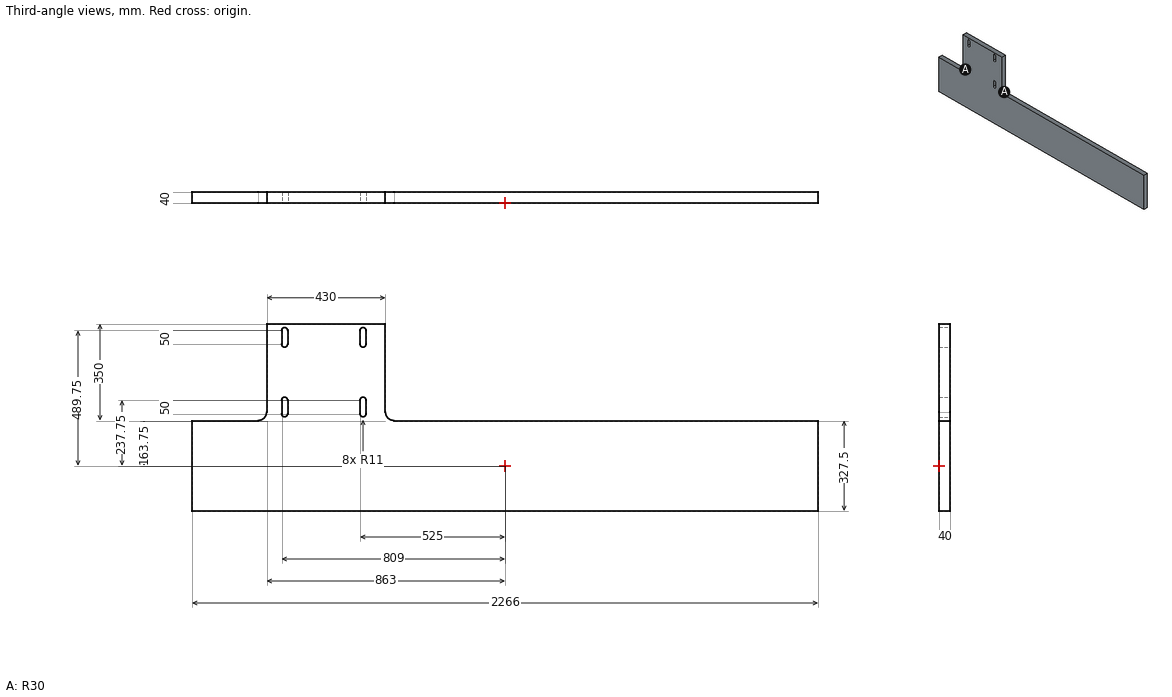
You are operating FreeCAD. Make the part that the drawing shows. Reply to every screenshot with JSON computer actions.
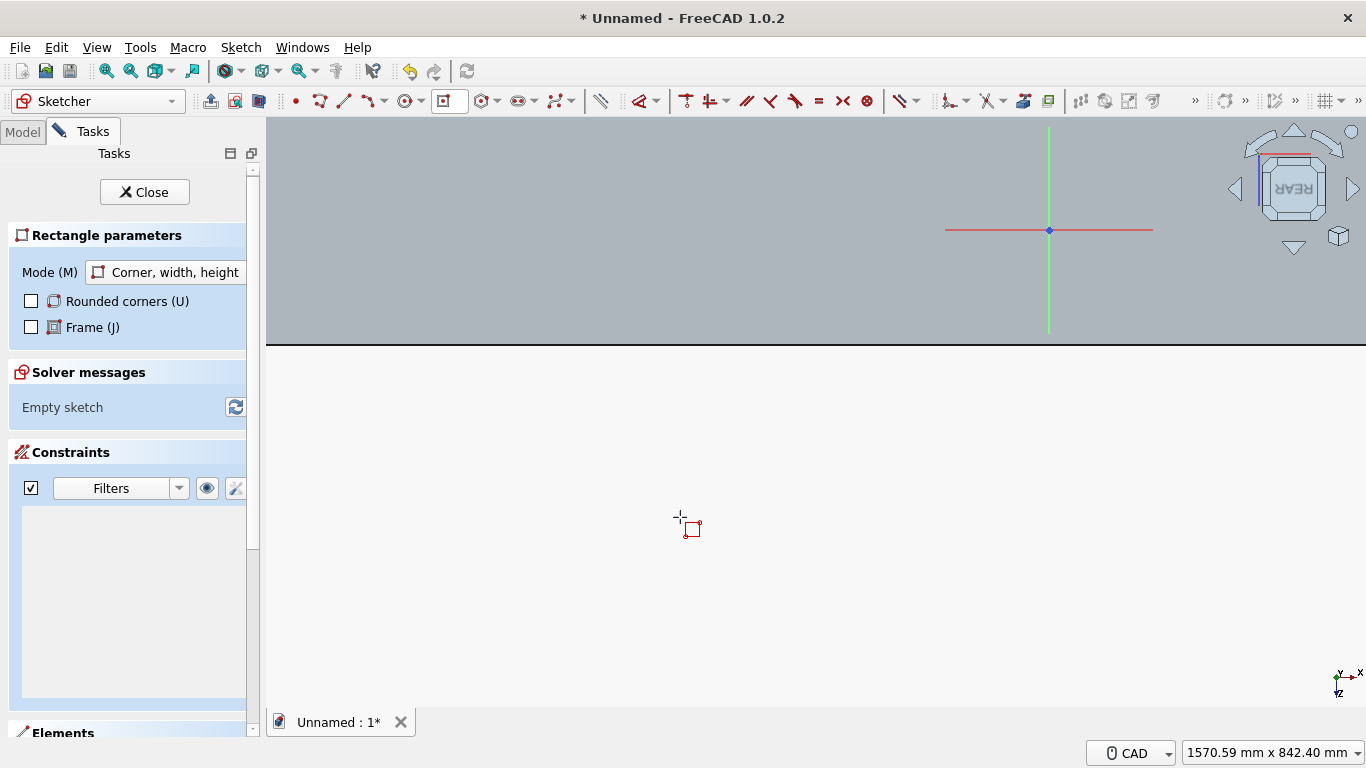
{"action": "left_click", "coordinate": [445, 345]}
{"action": "mouse_move", "coordinate": [746, 590]}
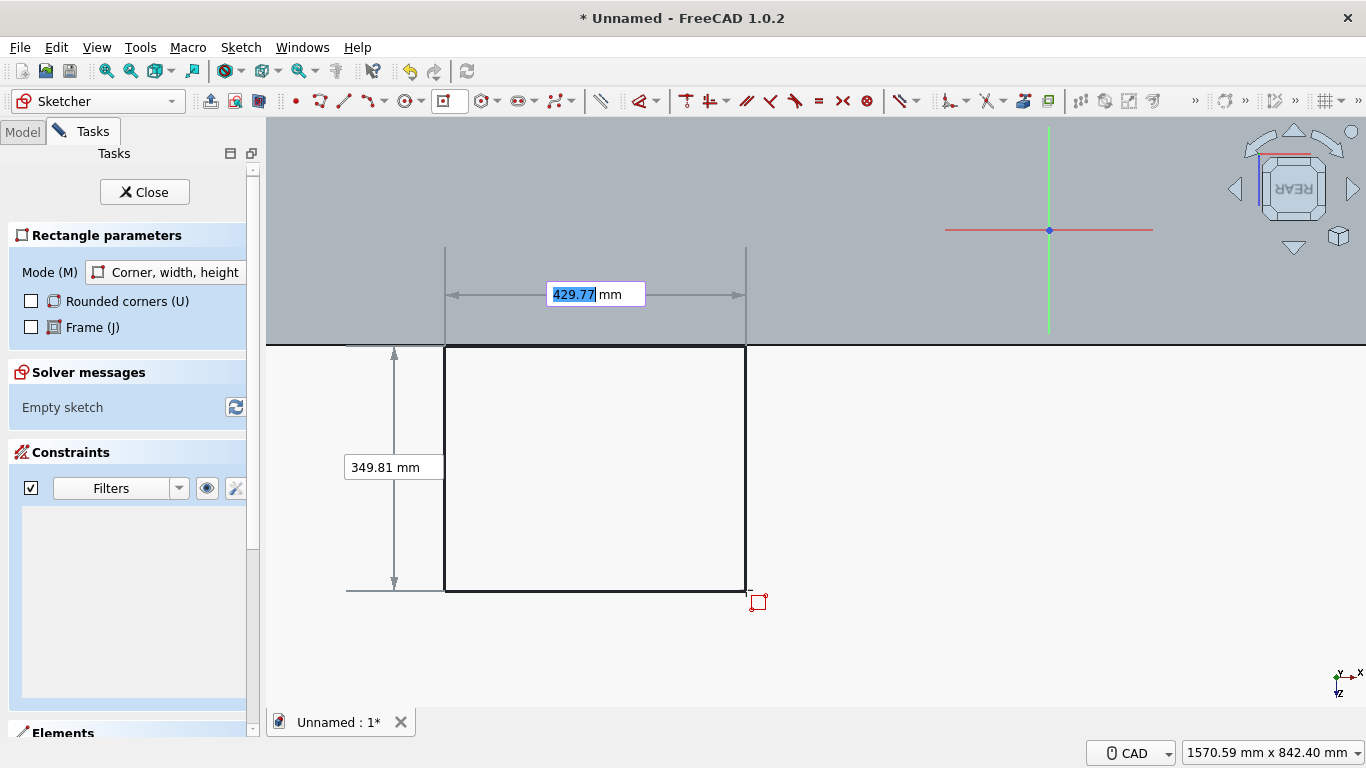
{"action": "type", "text": "430"}
{"action": "key", "text": "Tab"}
{"action": "type", "text": "350"}
{"action": "key", "text": "Return"}
{"action": "key", "text": "Escape"}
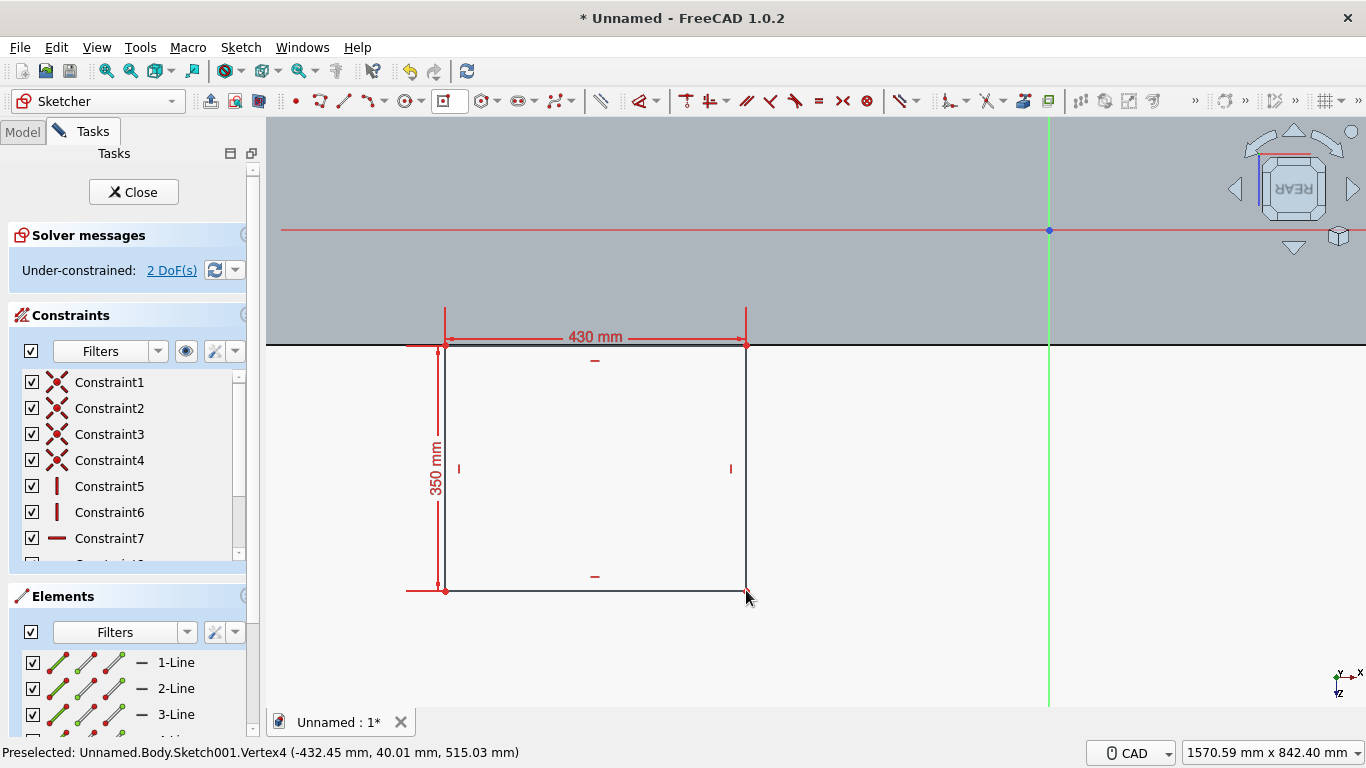
{"action": "left_click", "coordinate": [640, 102]}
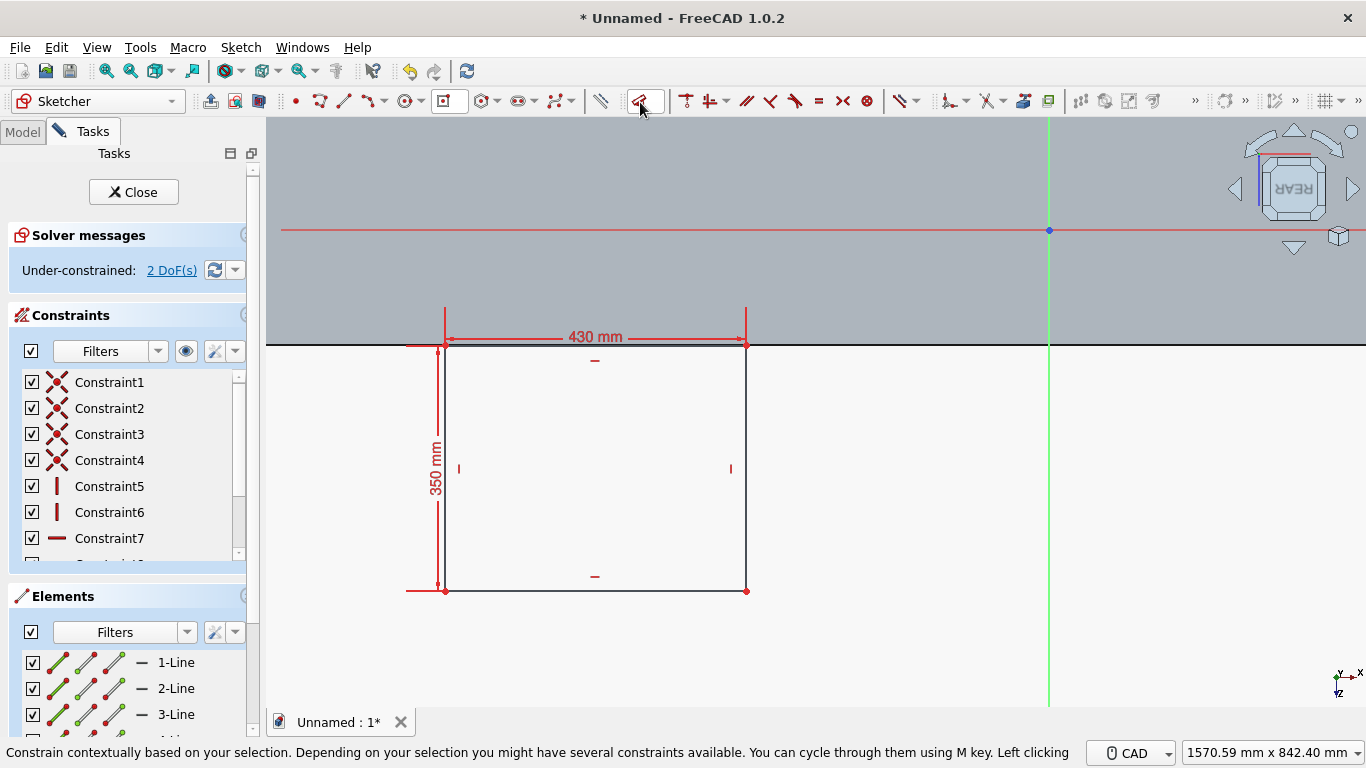
{"action": "left_click", "coordinate": [445, 346]}
{"action": "left_click", "coordinate": [747, 196]}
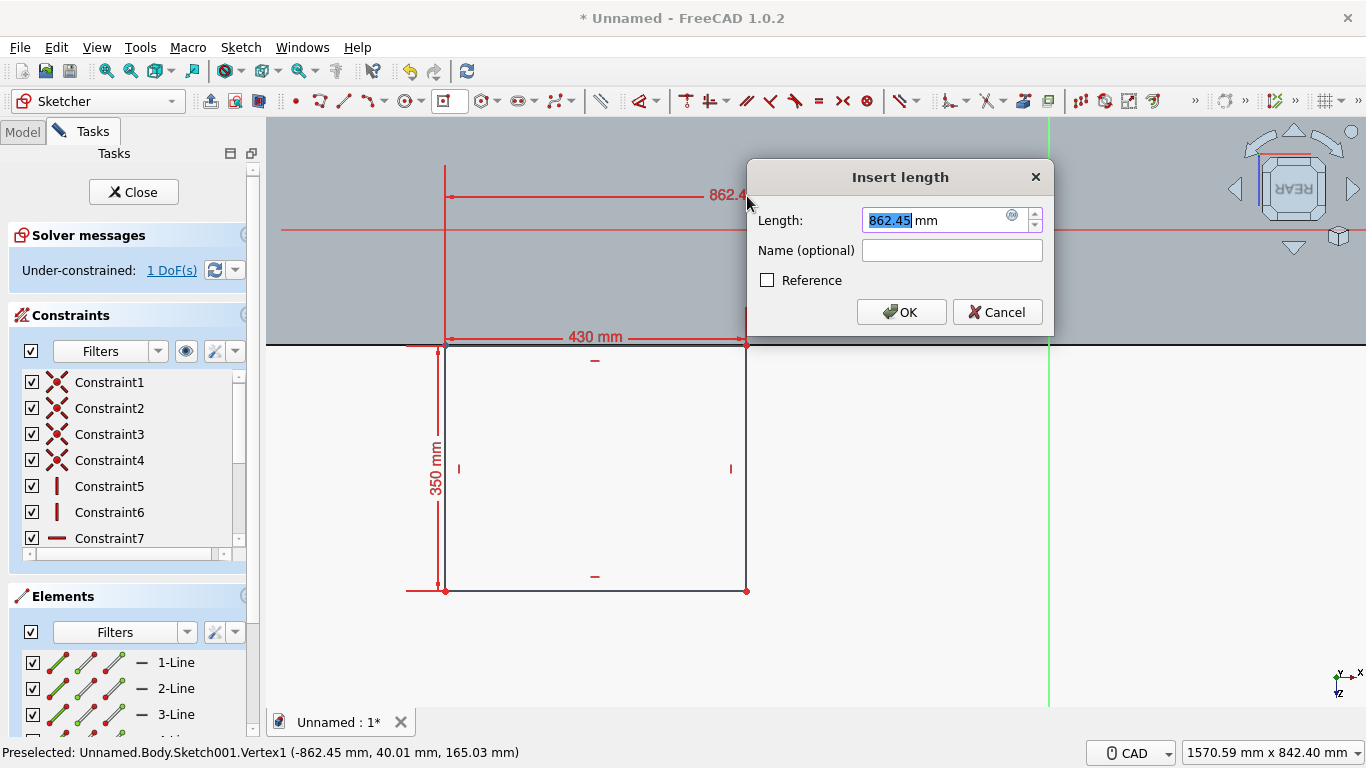
{"action": "type", "text": "863"}
{"action": "key", "text": "Return"}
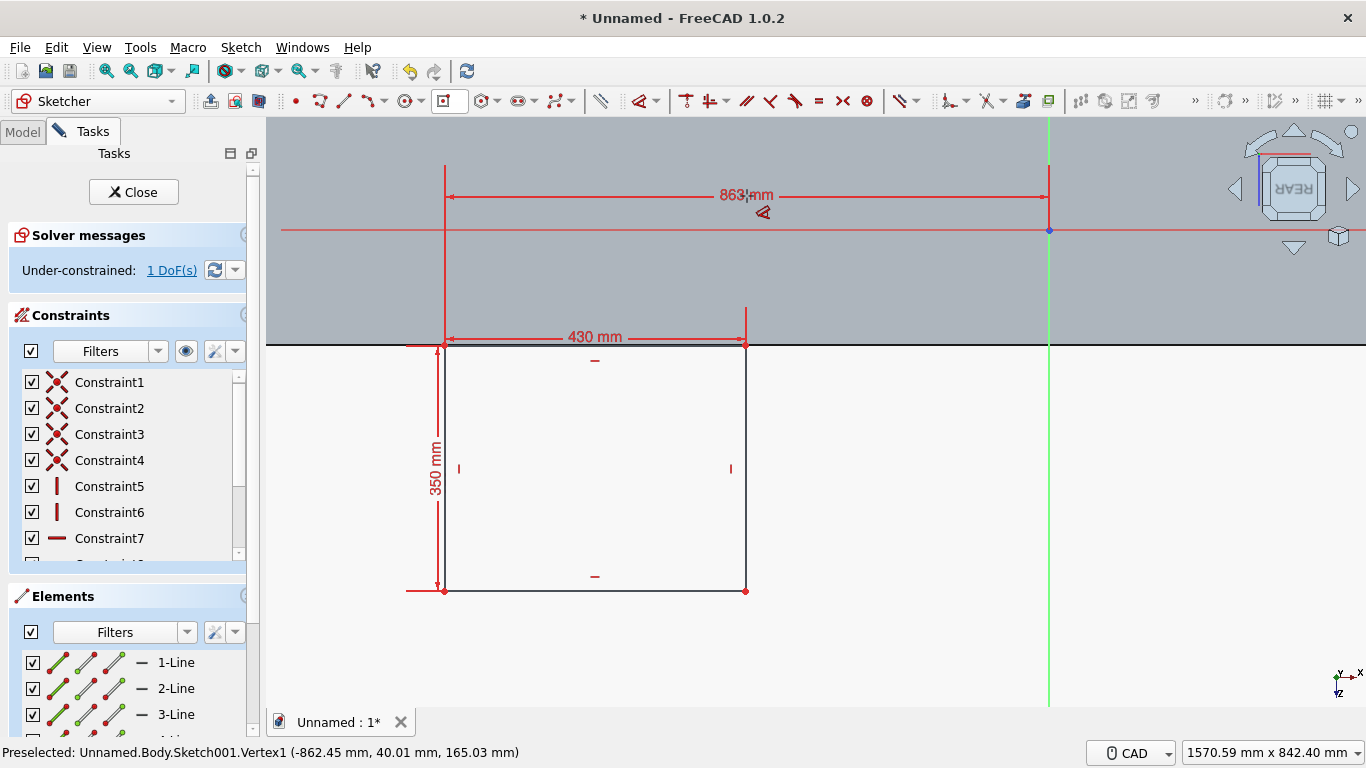
{"action": "left_click", "coordinate": [445, 346]}
{"action": "left_click", "coordinate": [1083, 288]}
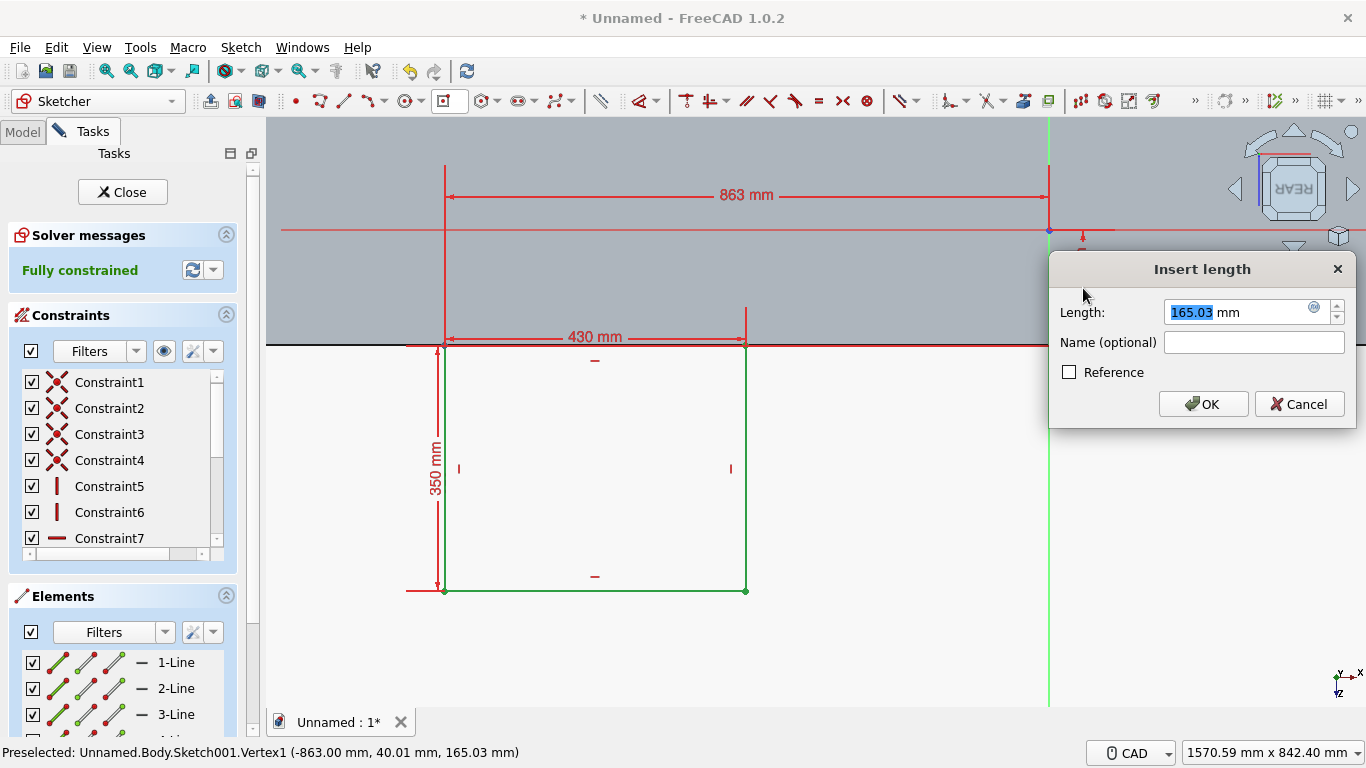
{"action": "type", "text": "163.75"}
{"action": "key", "text": "Return"}
{"action": "key", "text": "Escape"}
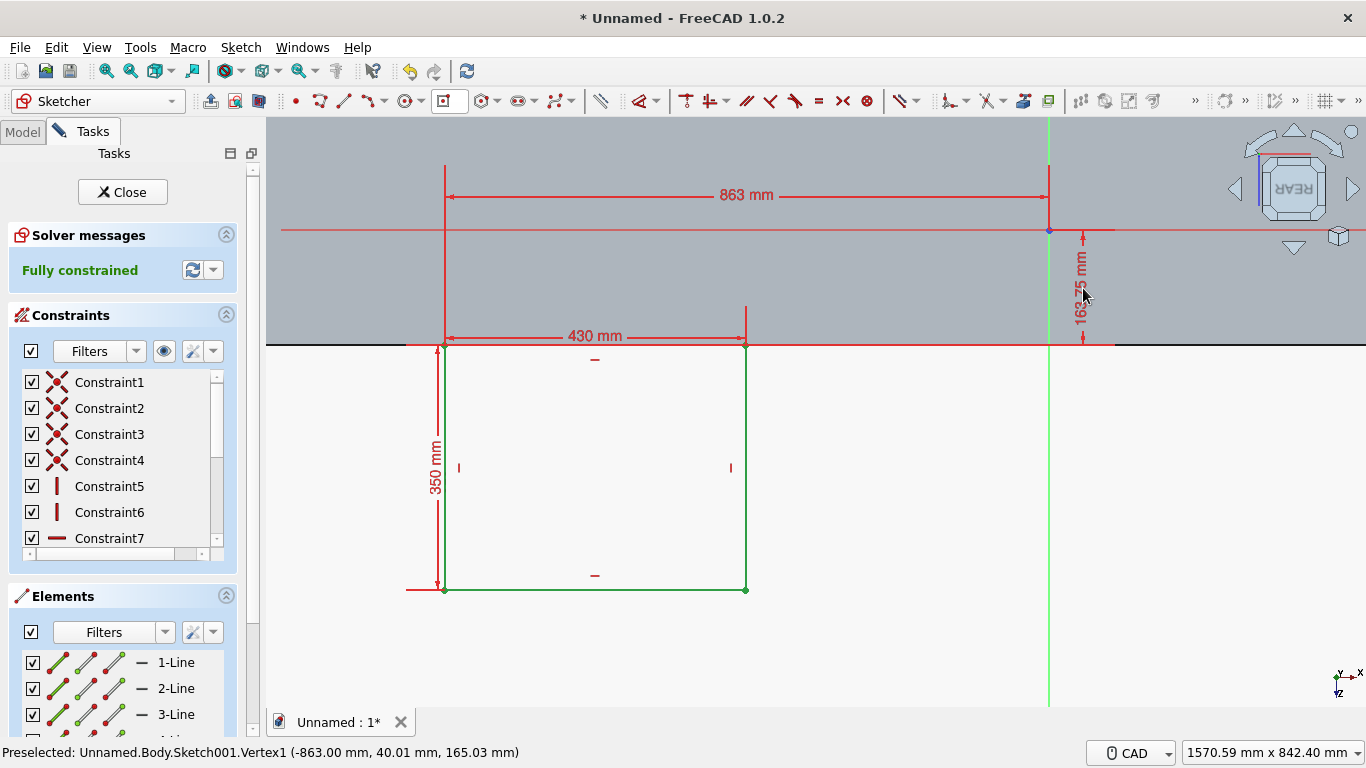
{"action": "left_click", "coordinate": [123, 192]}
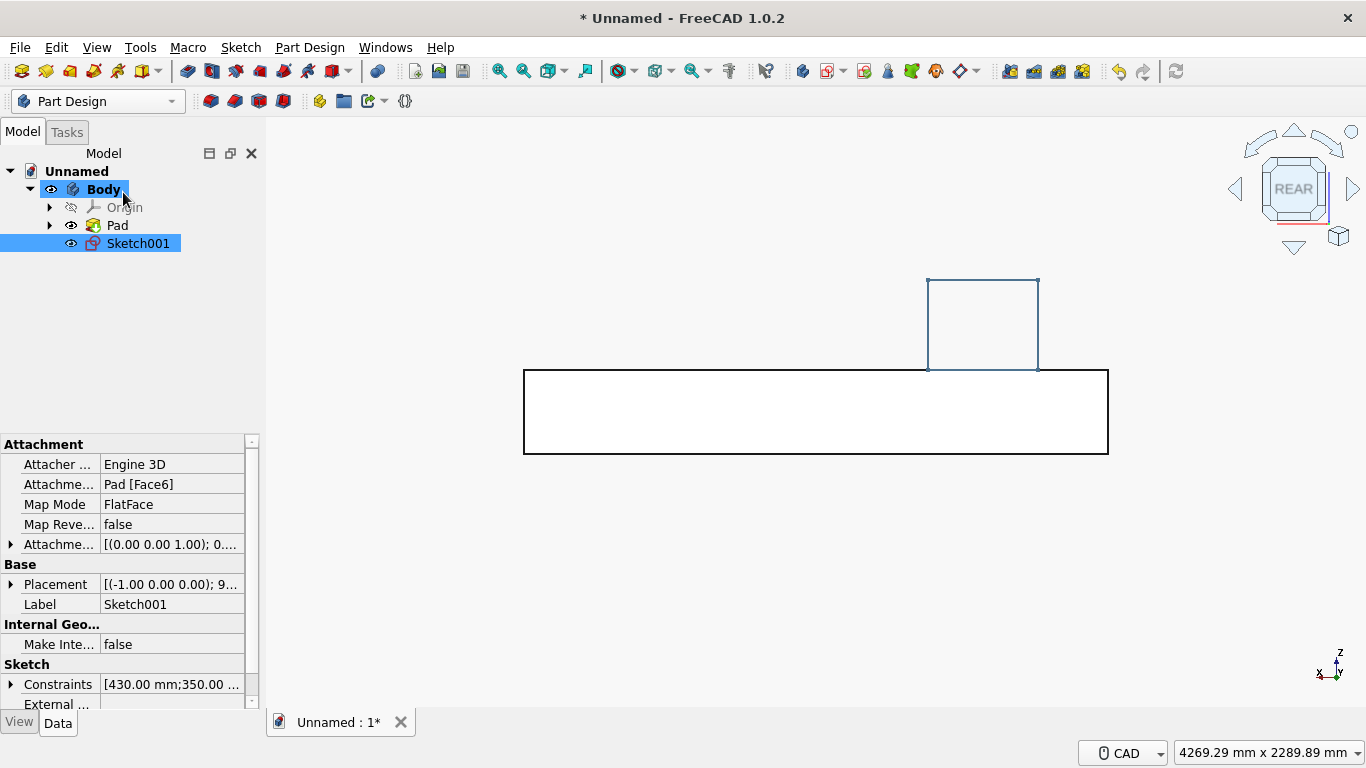
{"action": "left_click", "coordinate": [22, 72]}